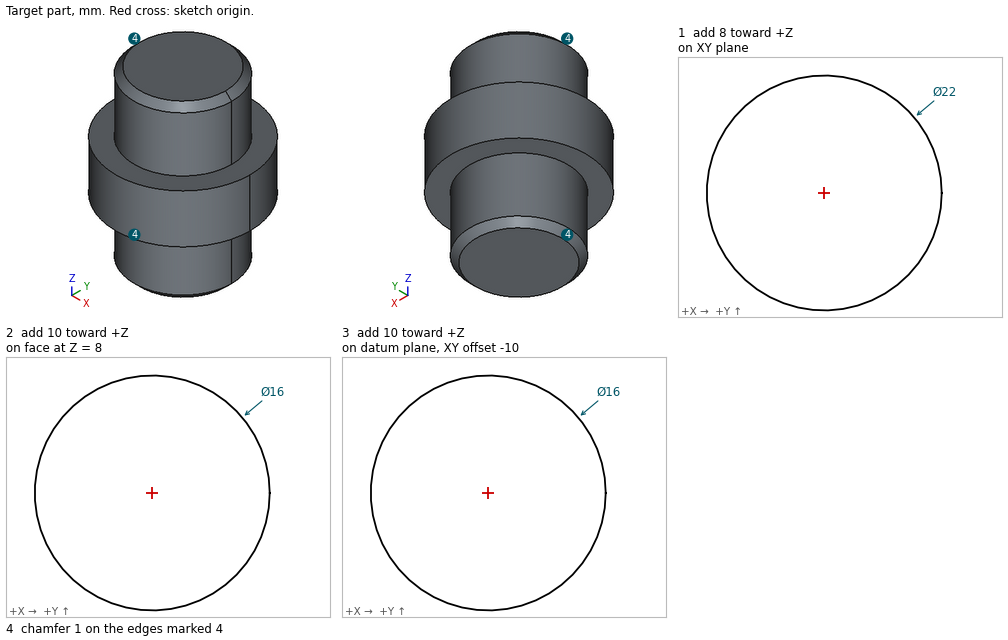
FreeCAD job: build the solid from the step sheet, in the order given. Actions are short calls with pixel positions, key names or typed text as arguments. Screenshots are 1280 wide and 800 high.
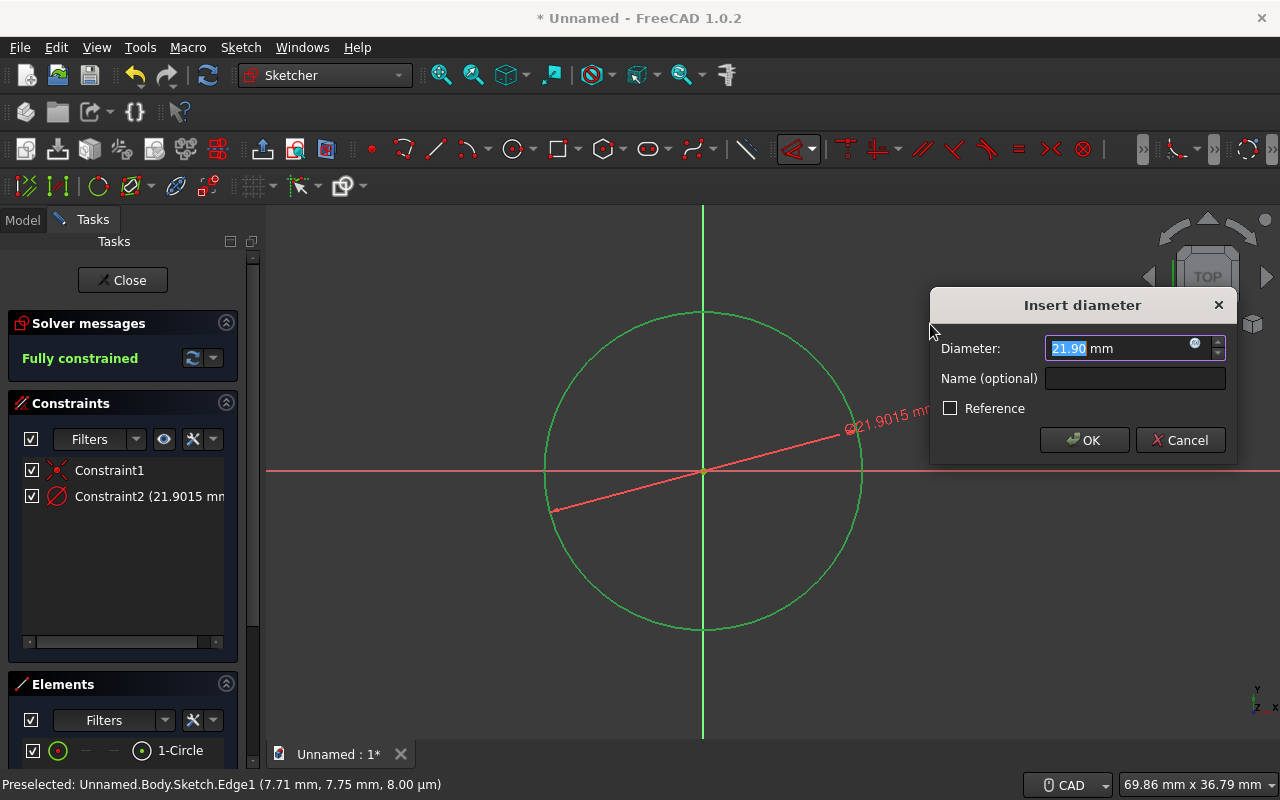
text(22)
key(Return)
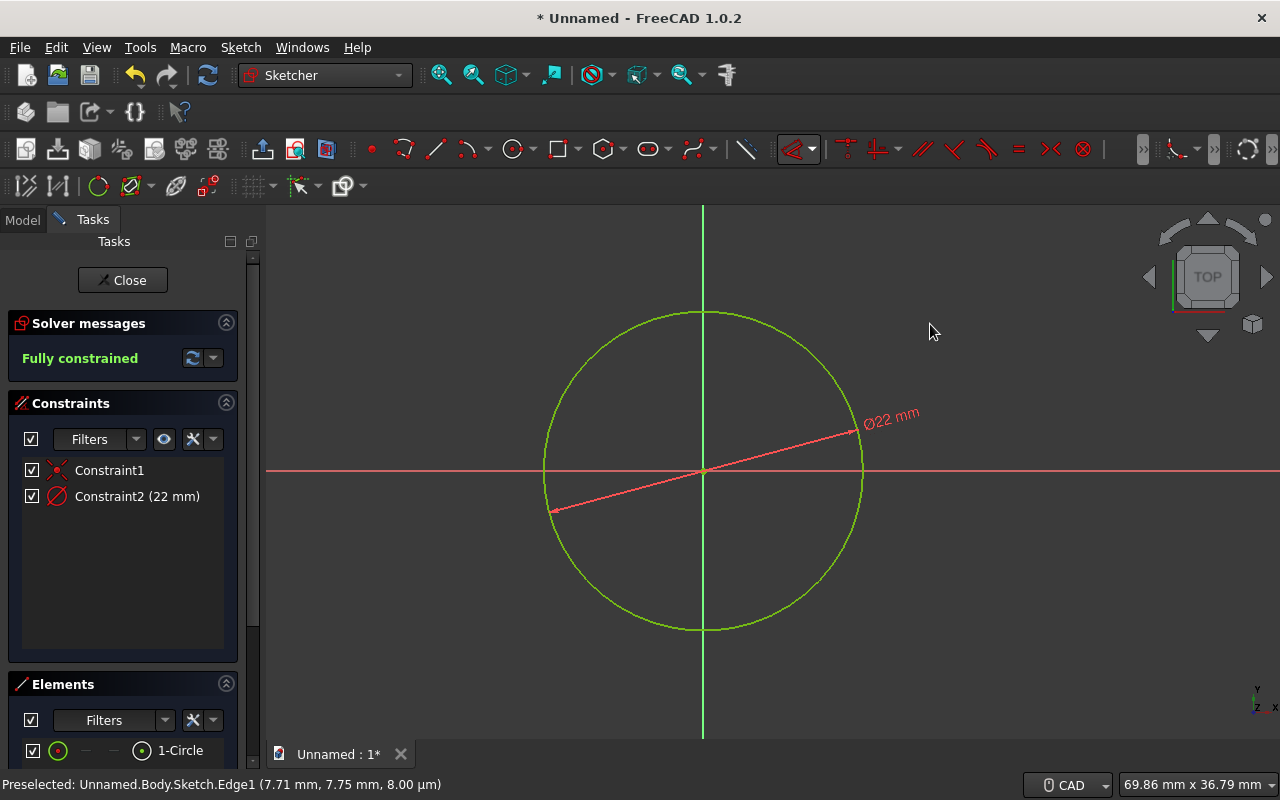
click(123, 280)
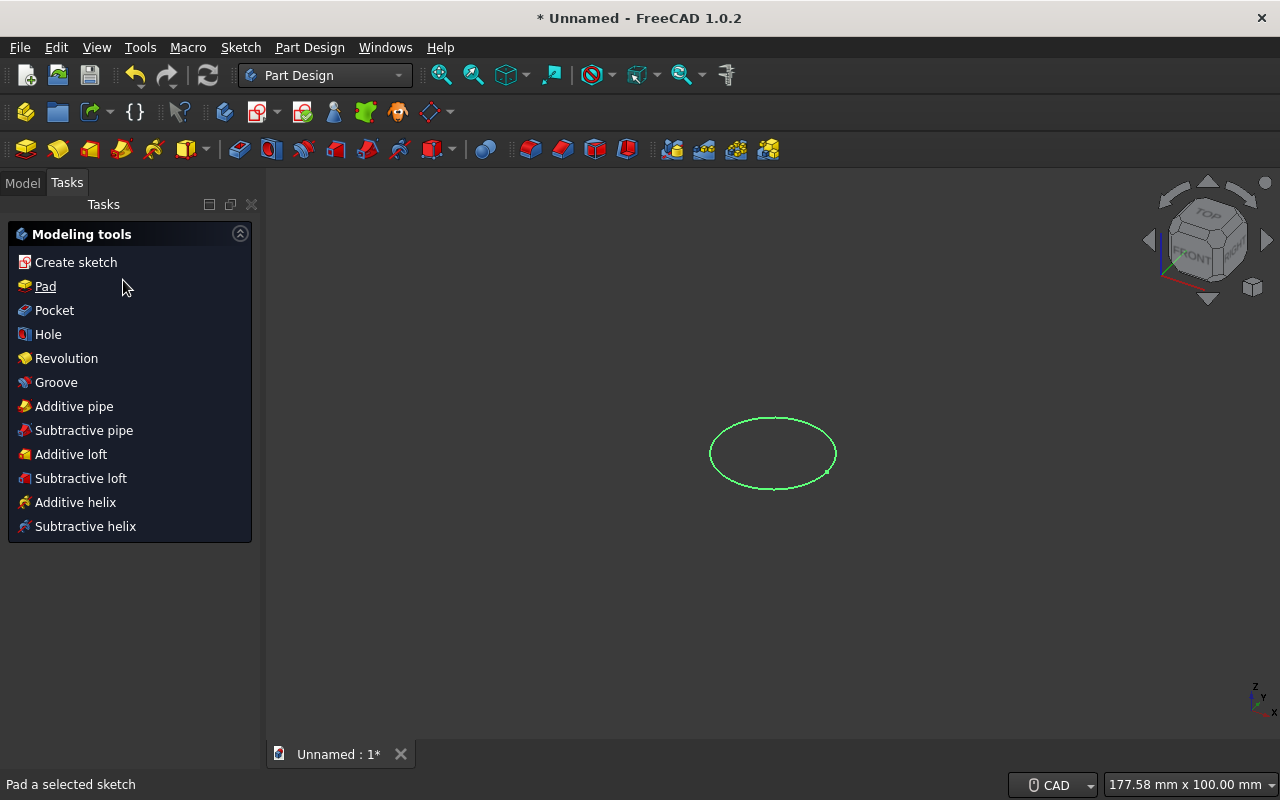
click(26, 150)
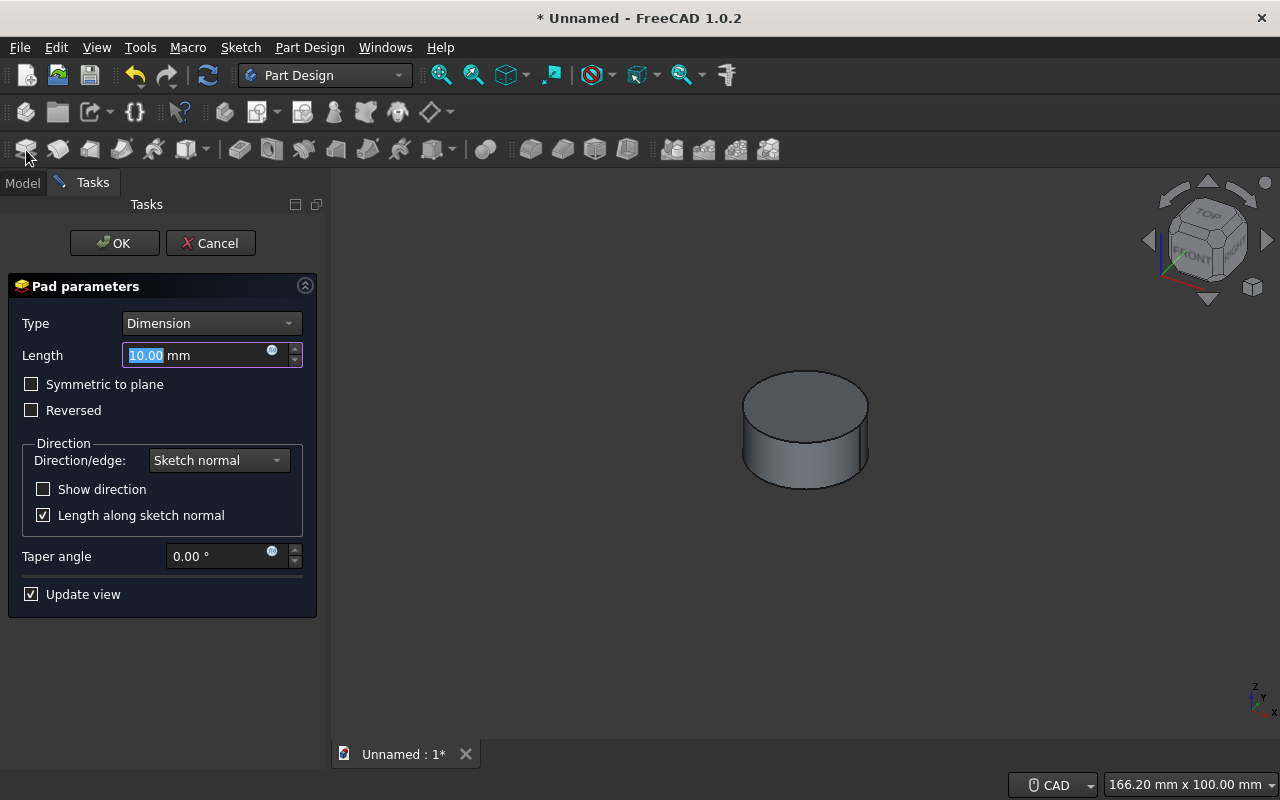
text(8)
key(Tab)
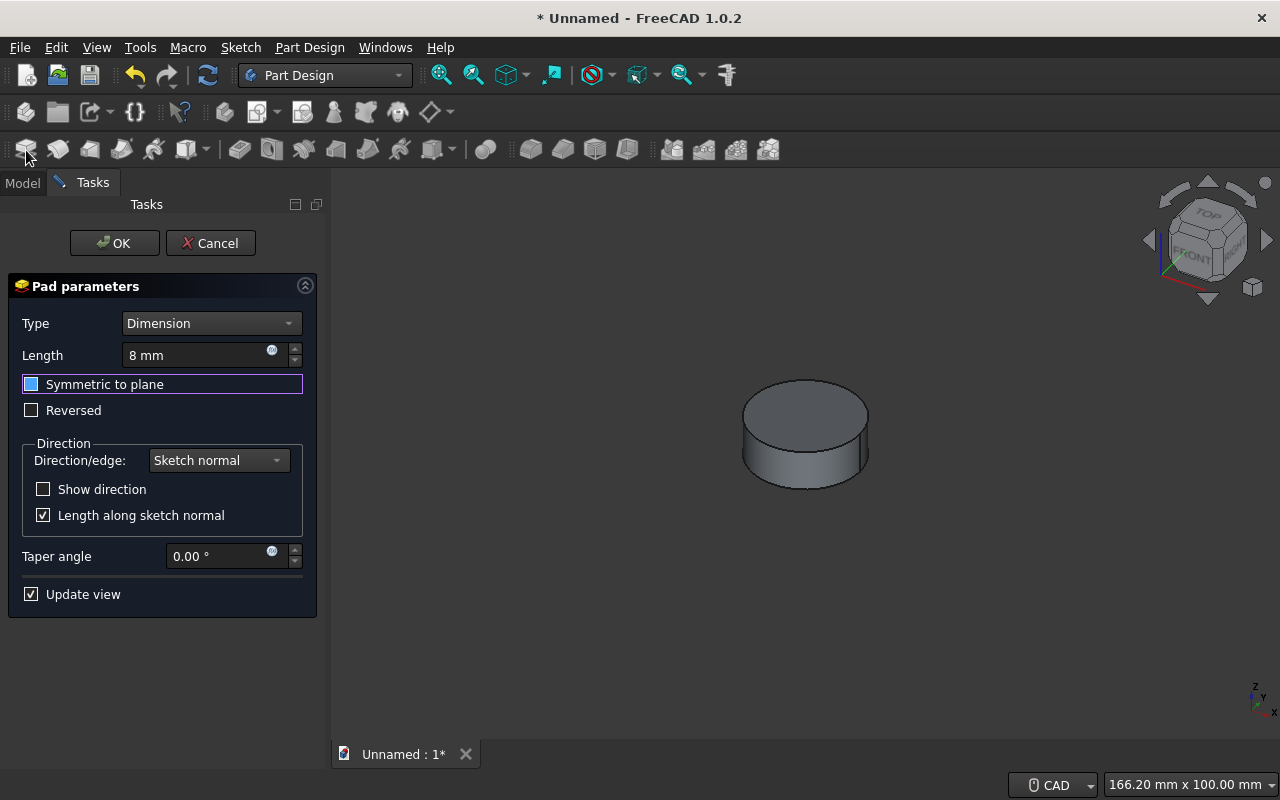
click(115, 243)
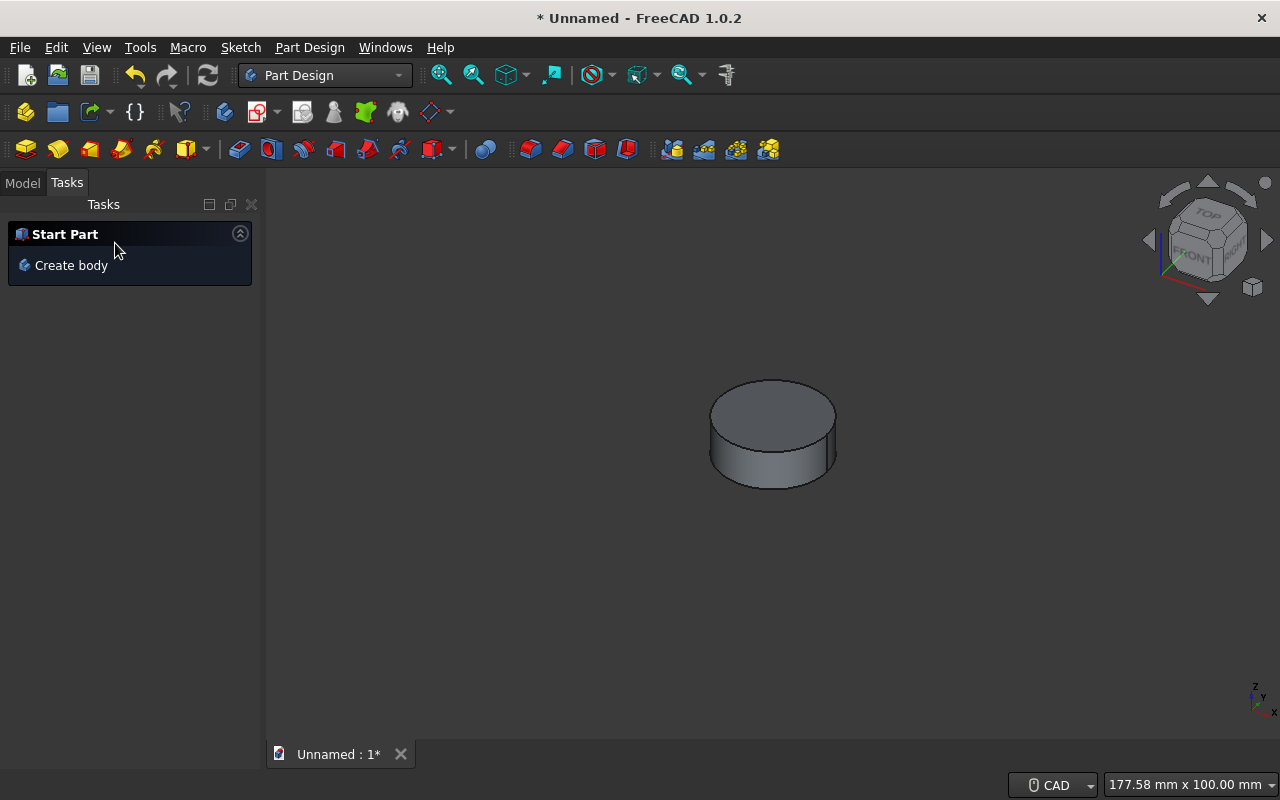
key(v)
key(f)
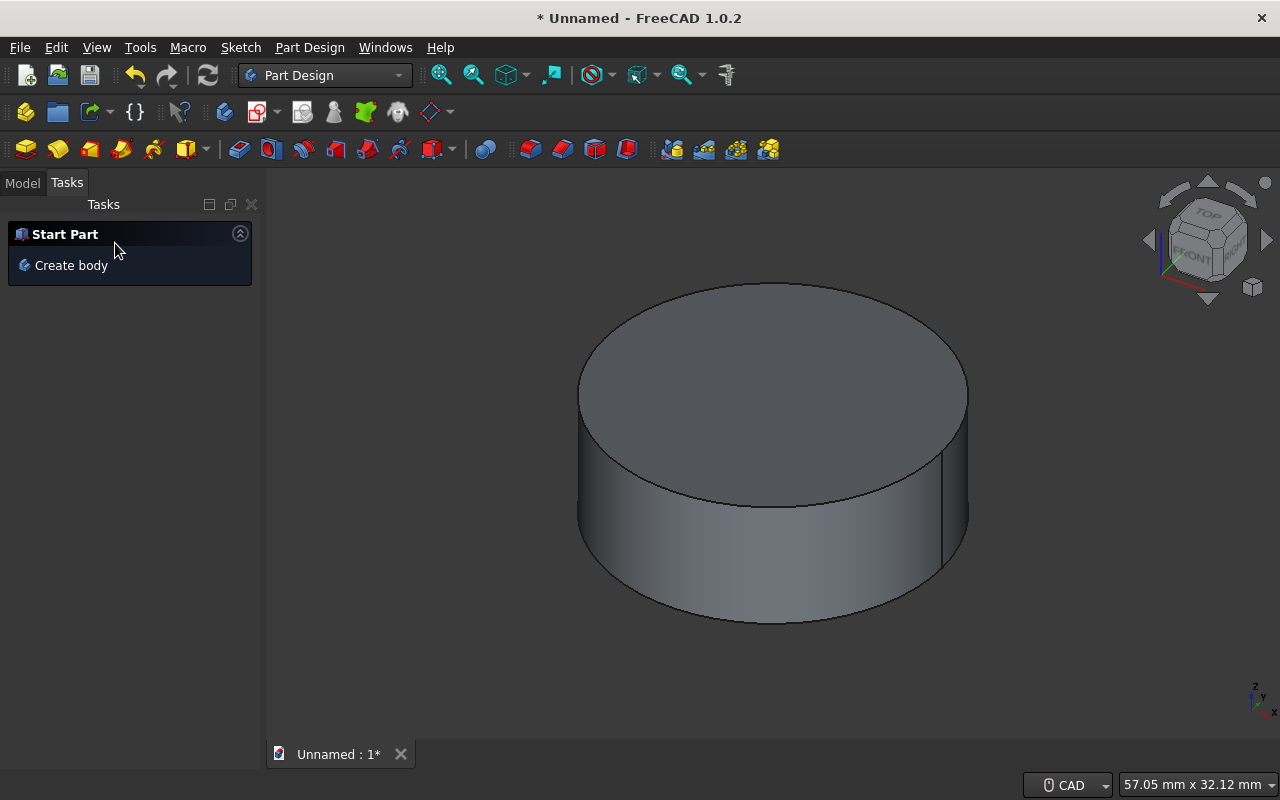
click(773, 394)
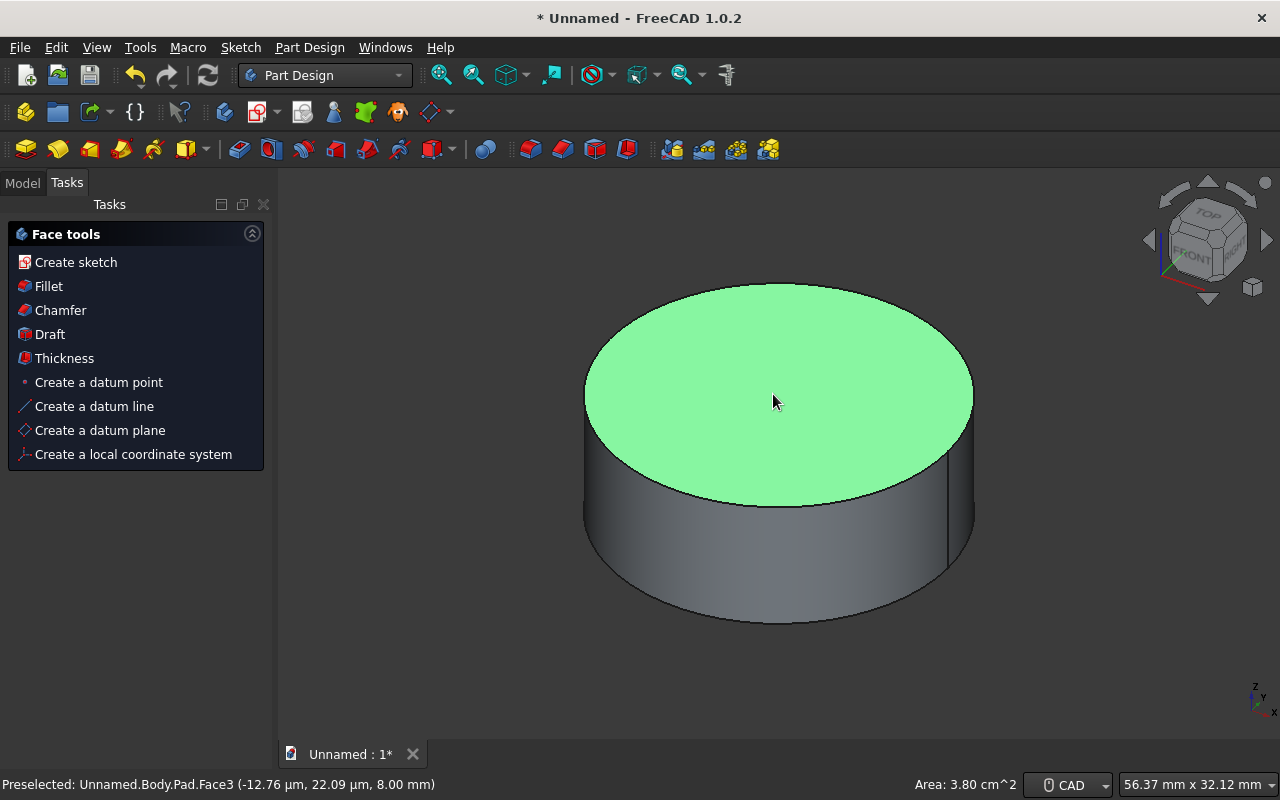
click(258, 112)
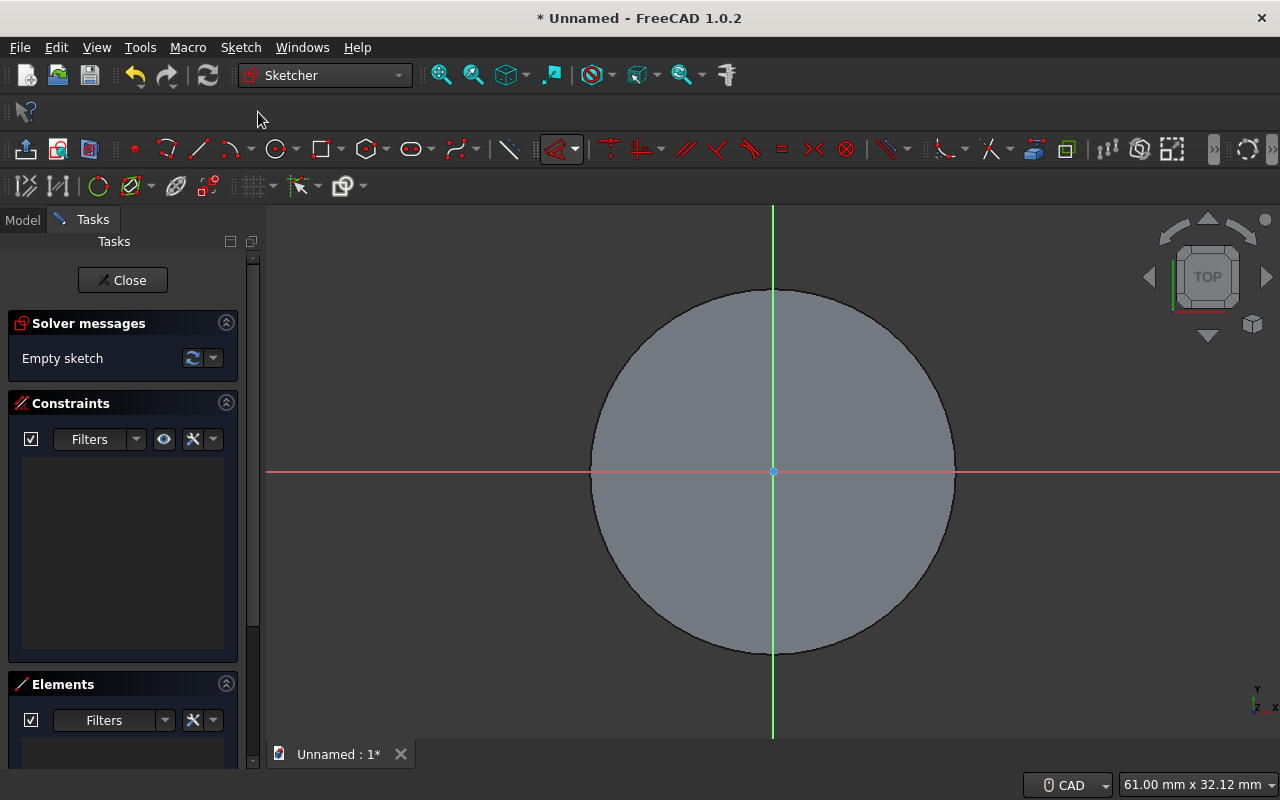
key(g)
key(c)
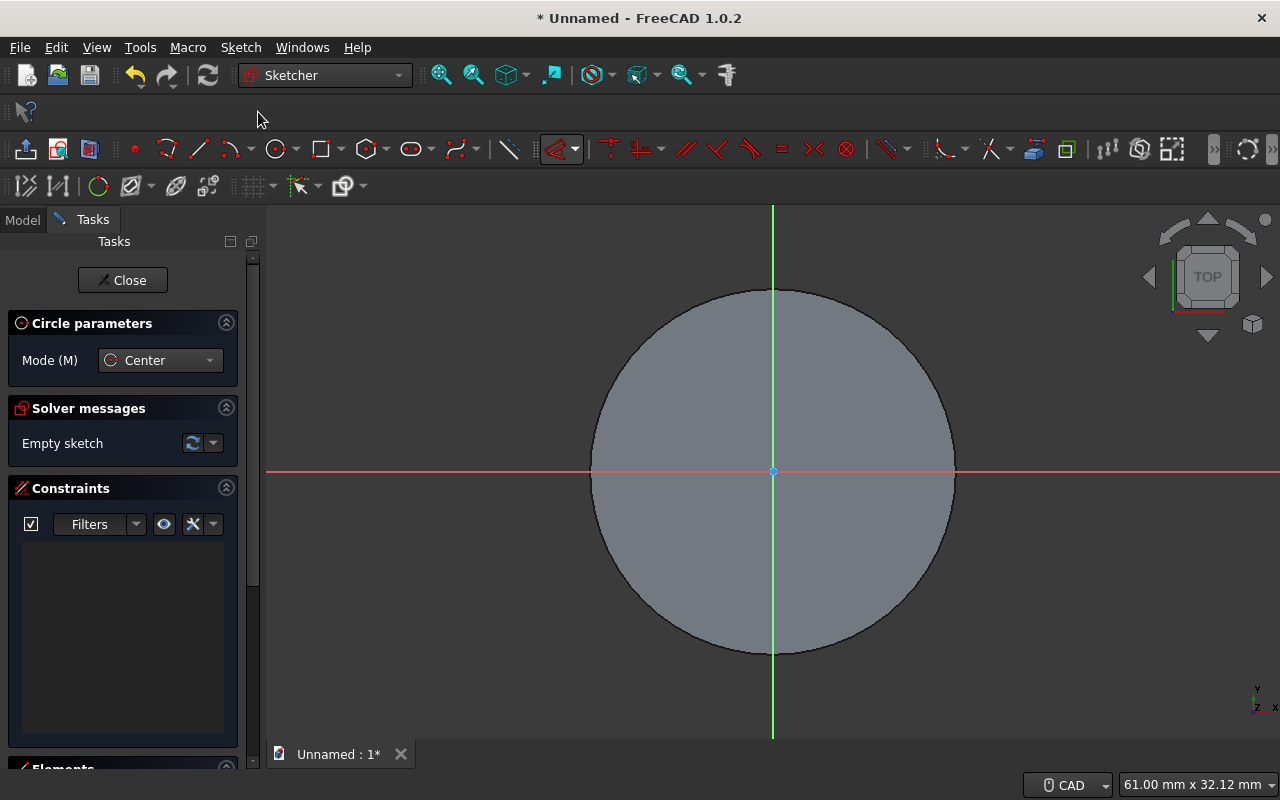
click(773, 472)
click(867, 378)
key(Escape)